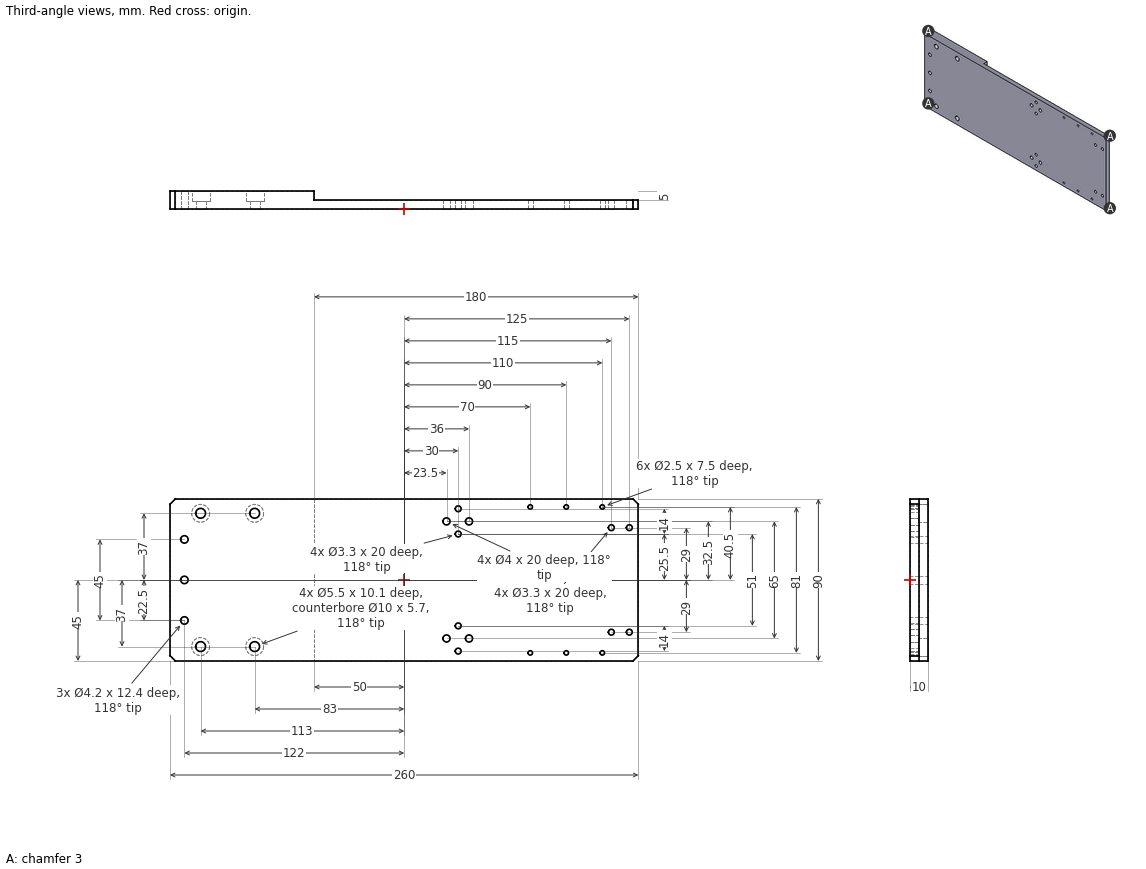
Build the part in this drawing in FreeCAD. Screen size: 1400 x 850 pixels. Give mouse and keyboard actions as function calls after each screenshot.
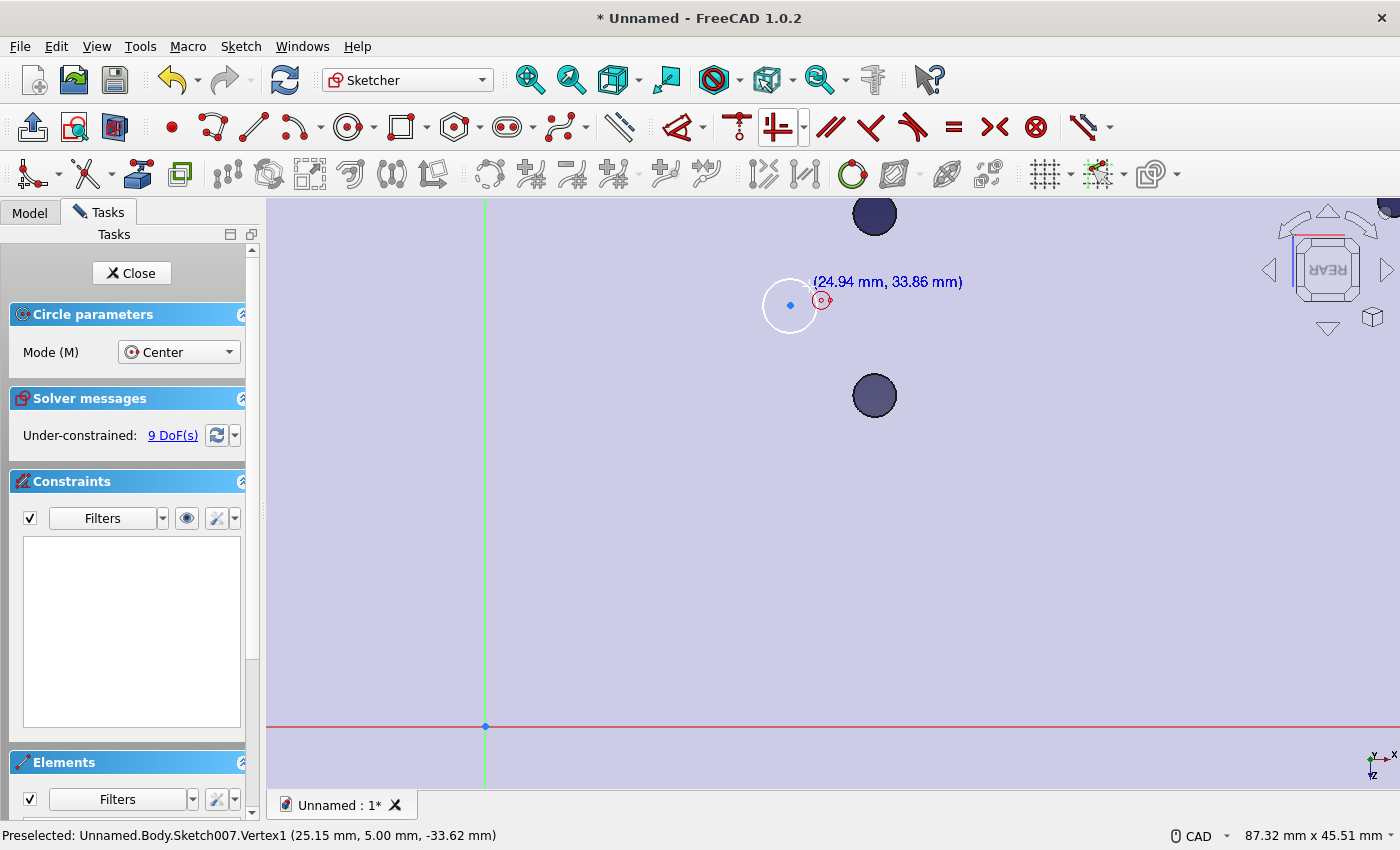
click(953, 305)
click(971, 286)
key(Escape)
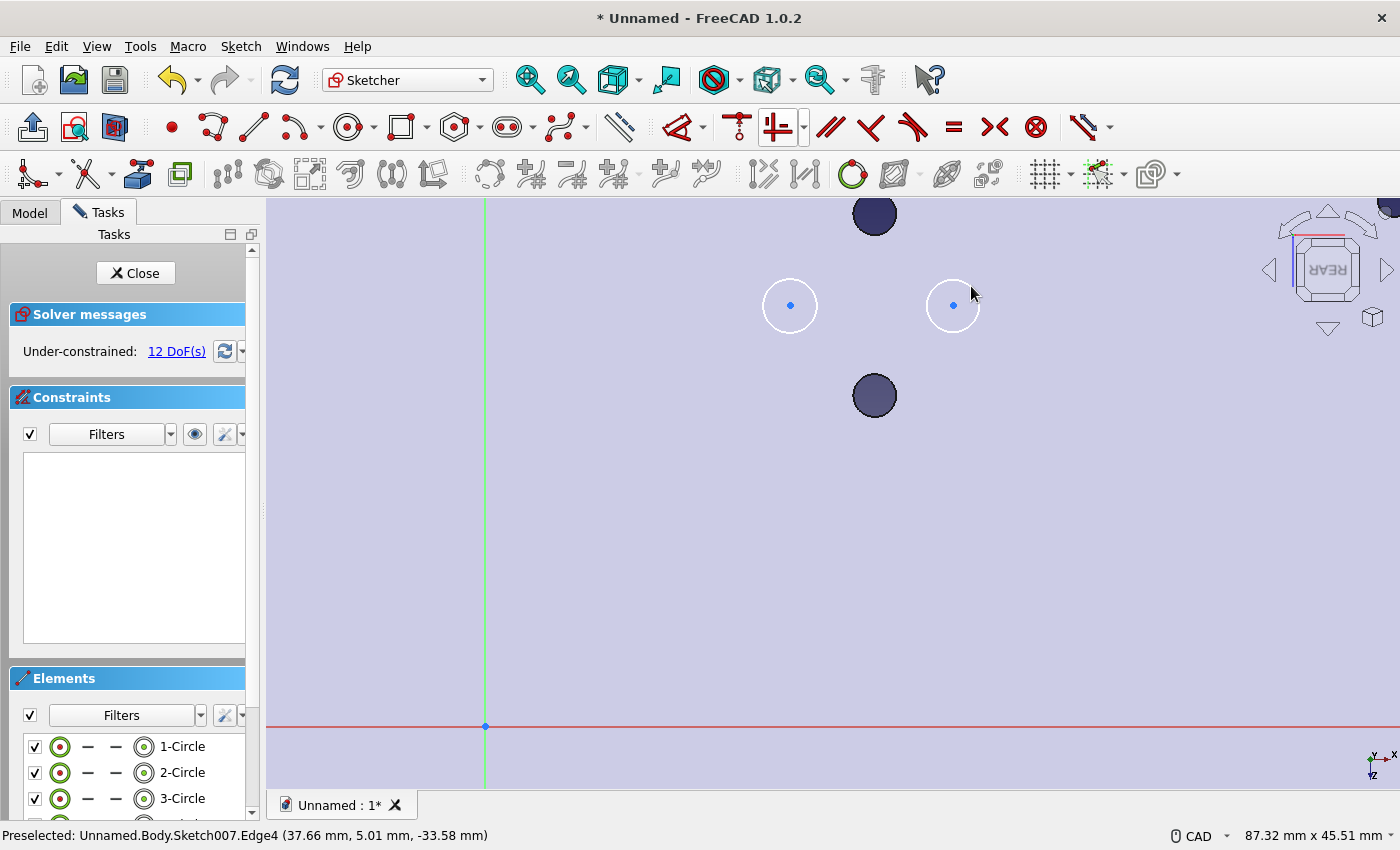
scroll(791, 303, down, 4)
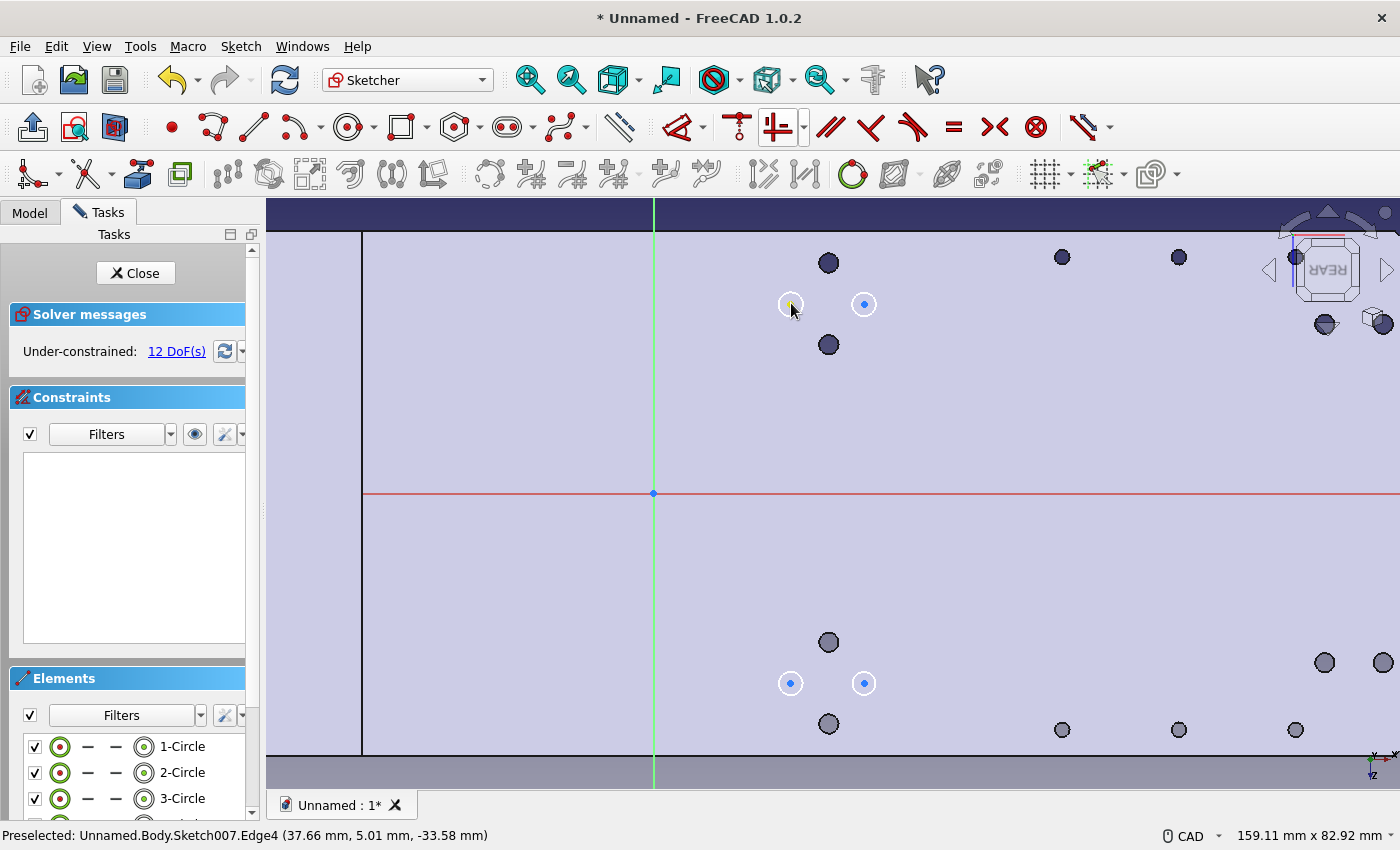
click(799, 675)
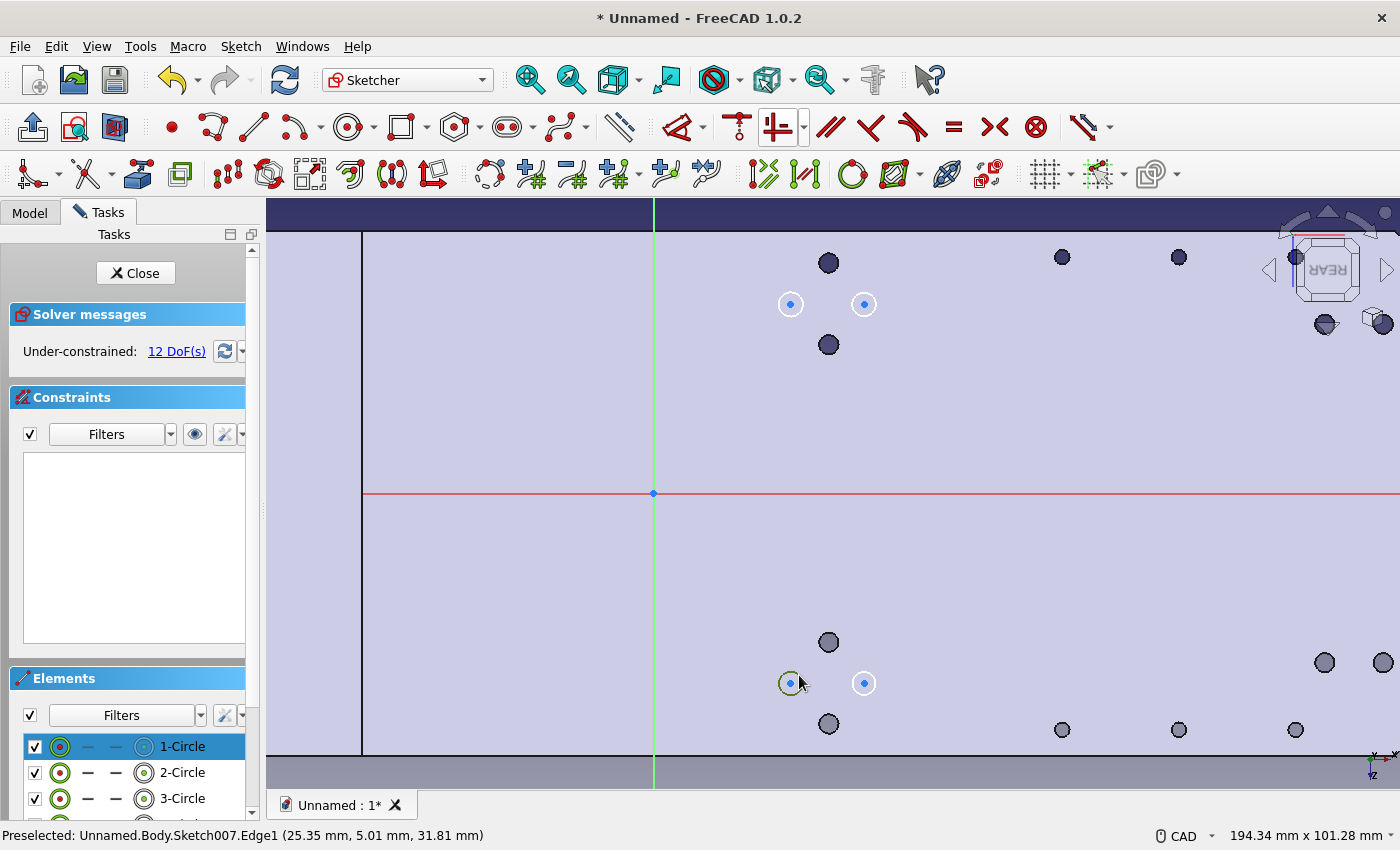
click(872, 675)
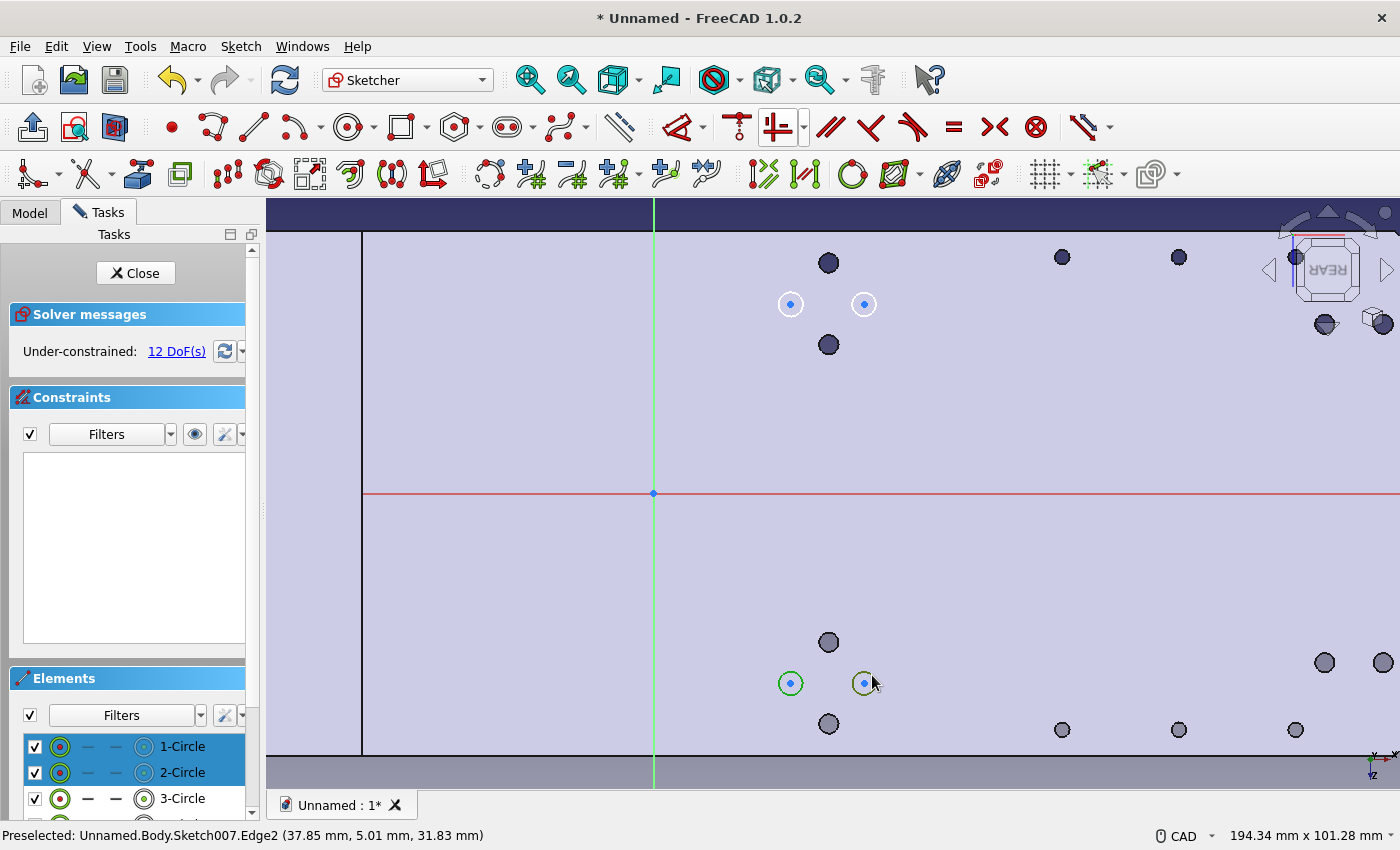
click(799, 296)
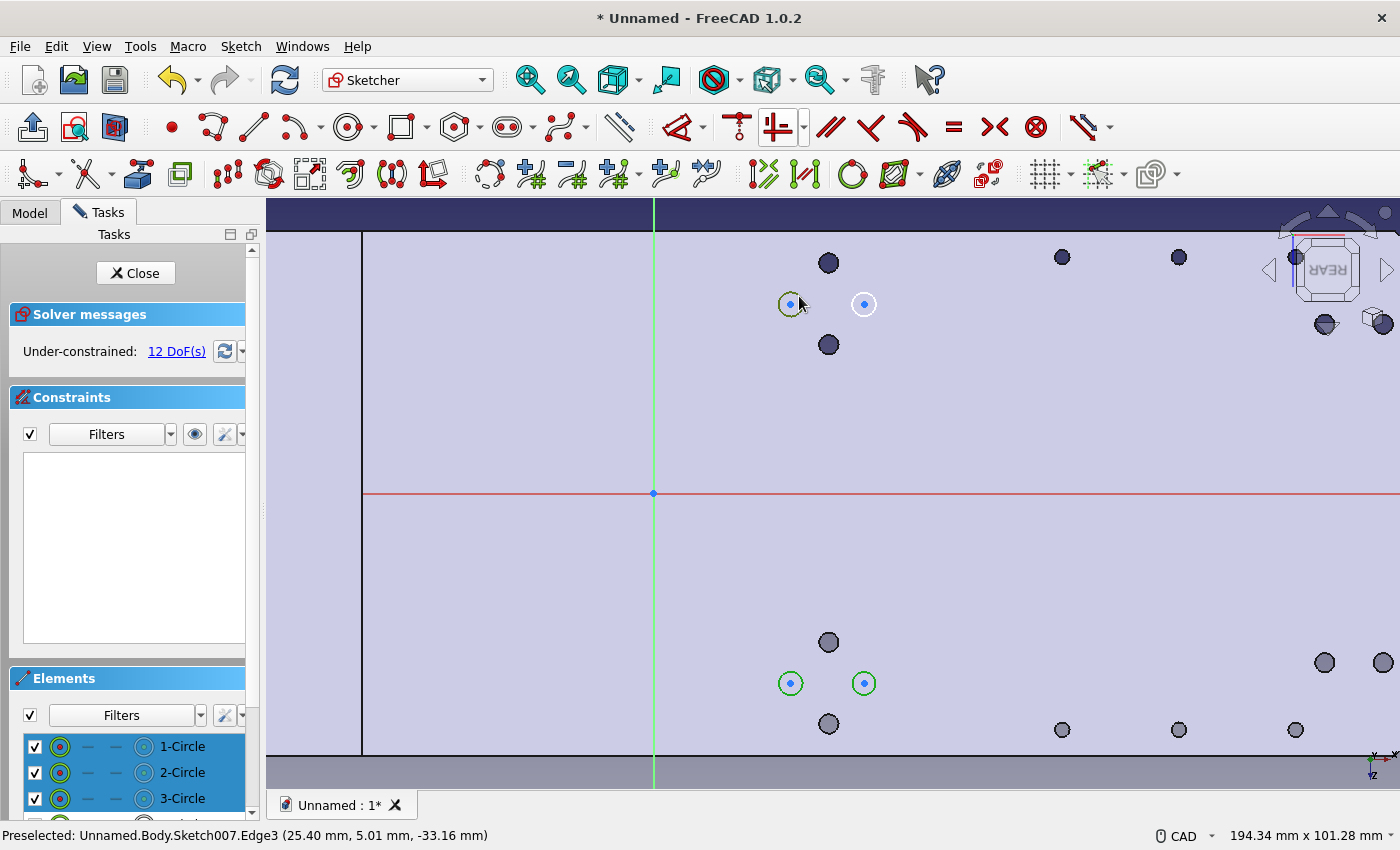
click(872, 296)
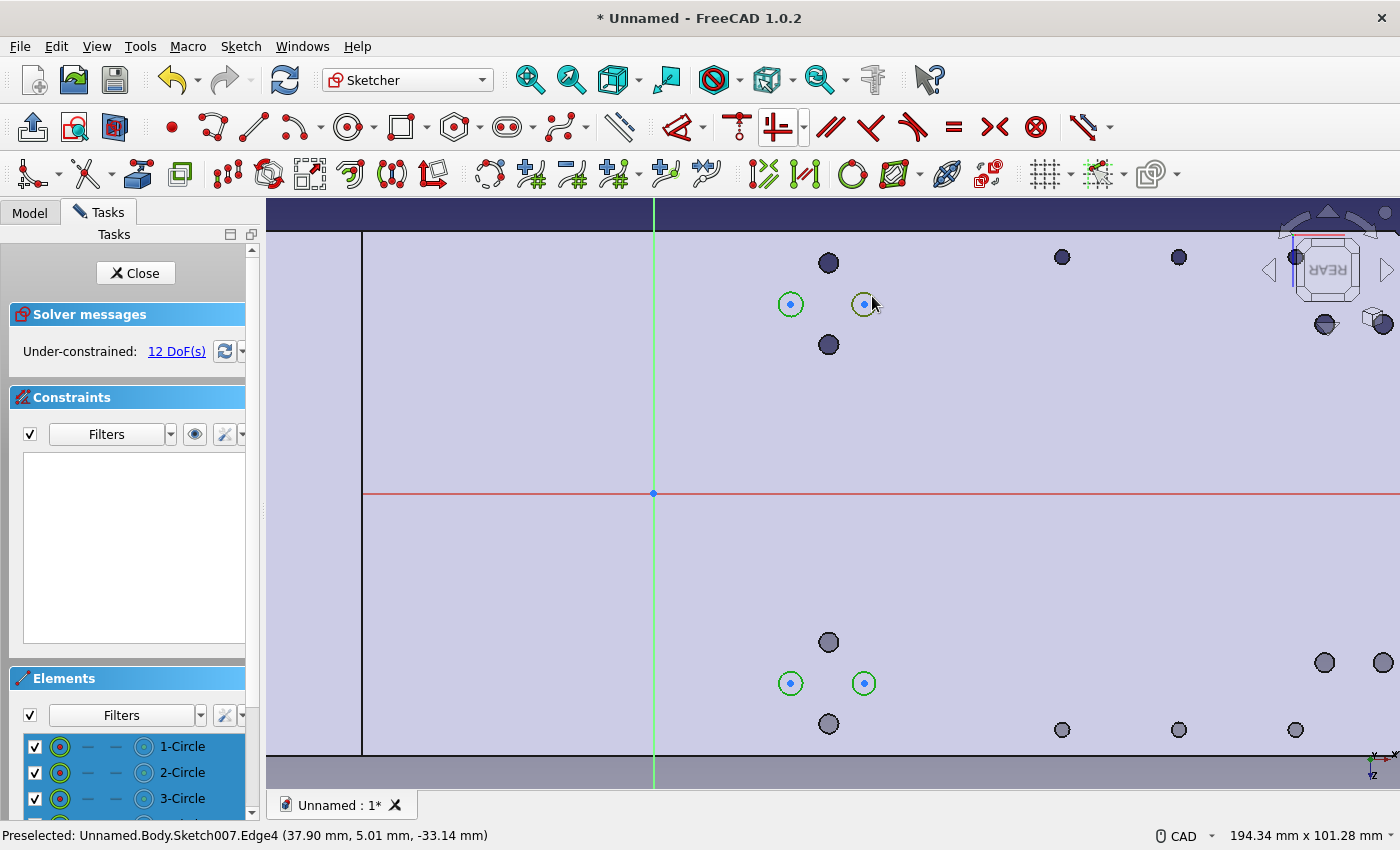
click(954, 128)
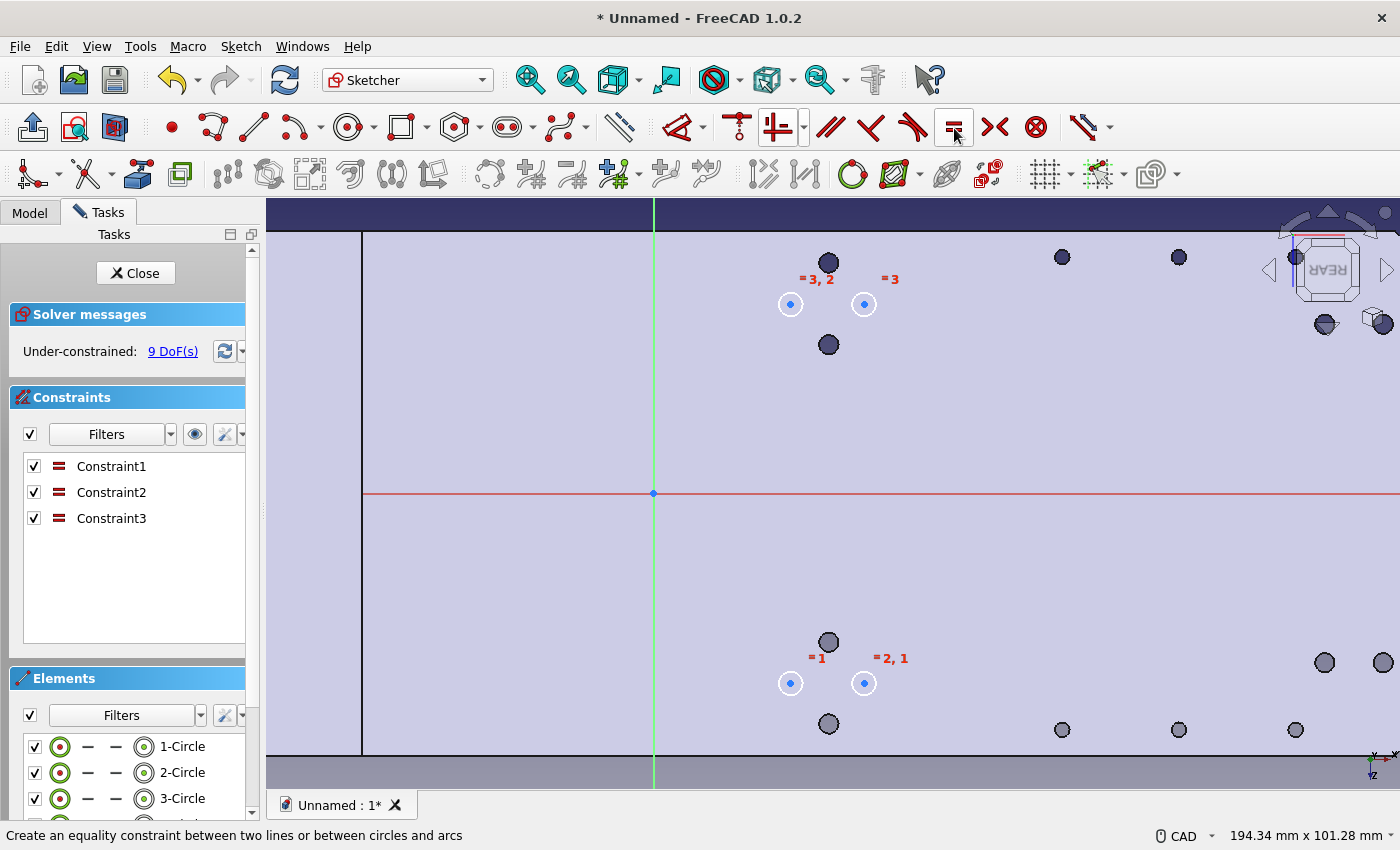
click(791, 683)